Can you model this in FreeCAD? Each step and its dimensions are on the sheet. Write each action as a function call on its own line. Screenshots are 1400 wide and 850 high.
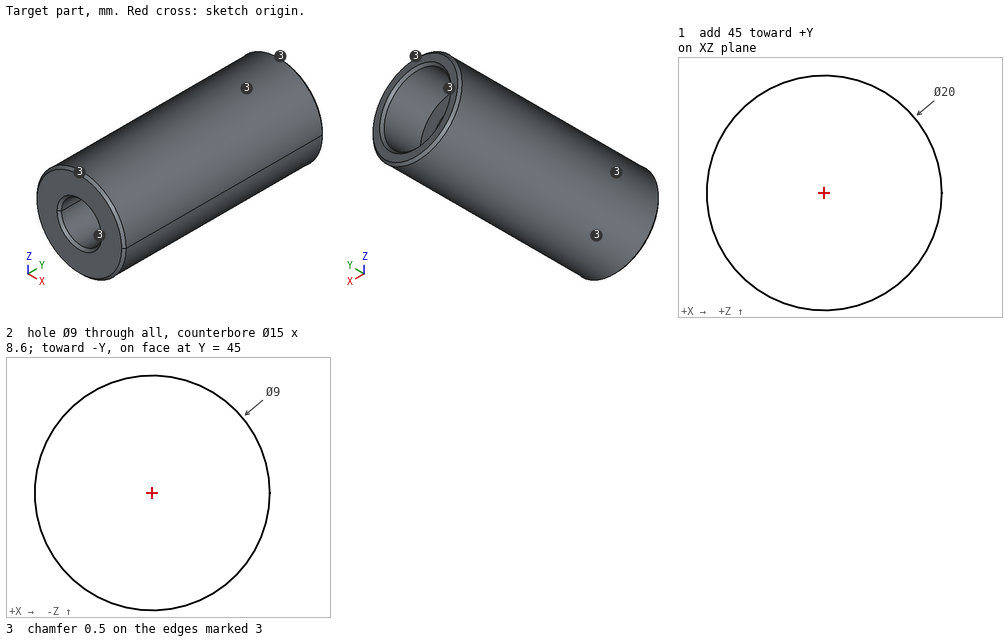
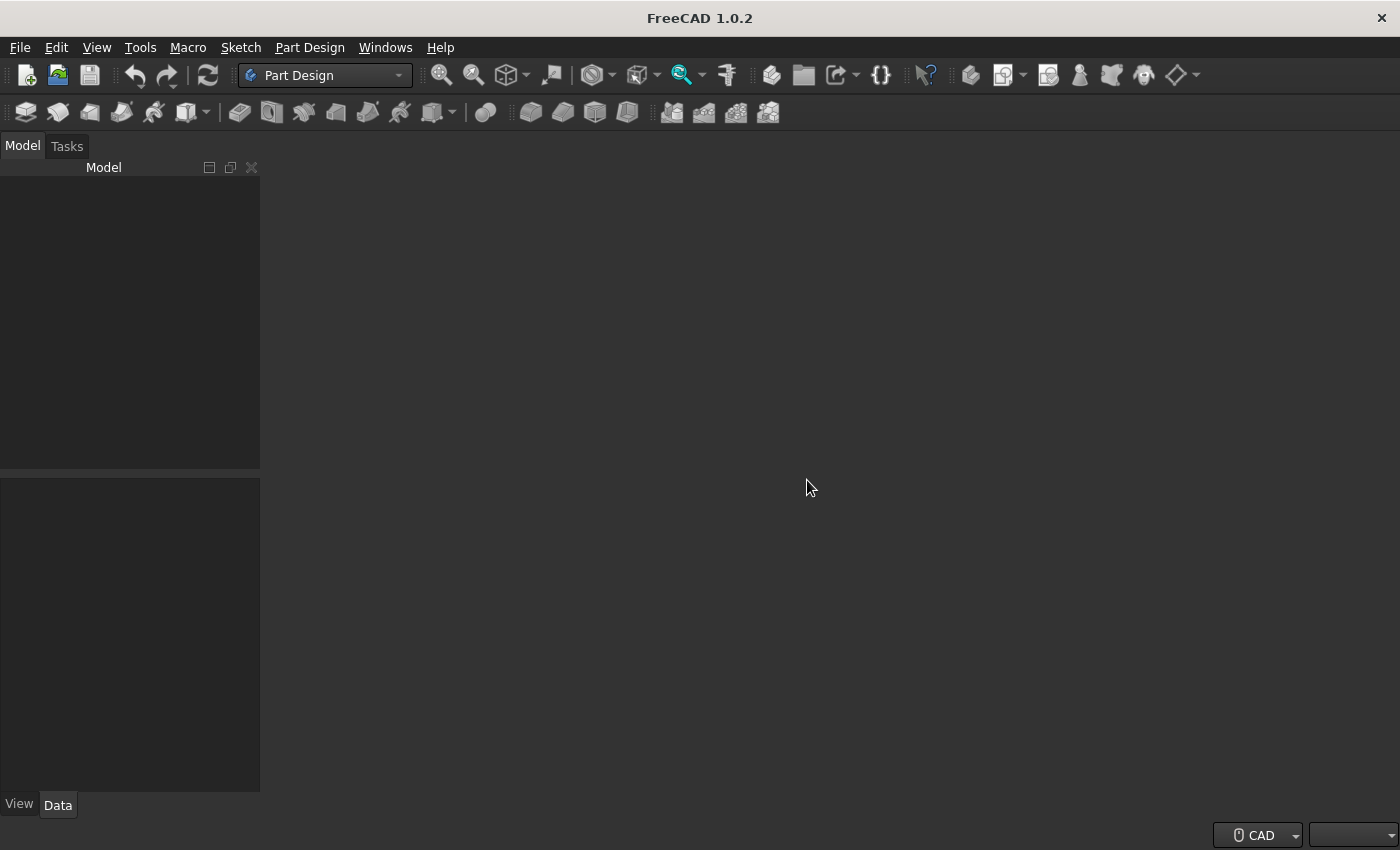
key(ctrl+n)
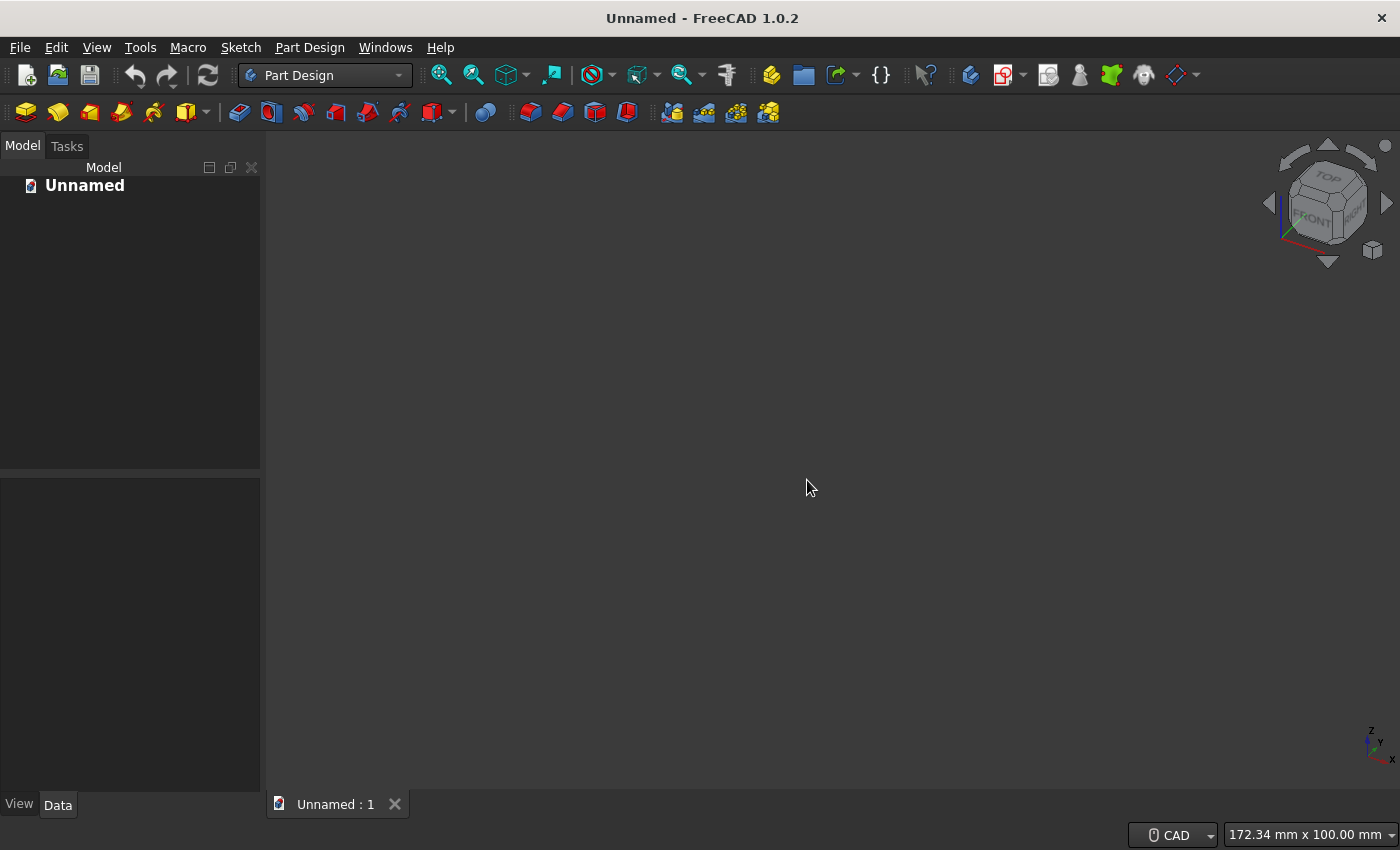
click(1004, 76)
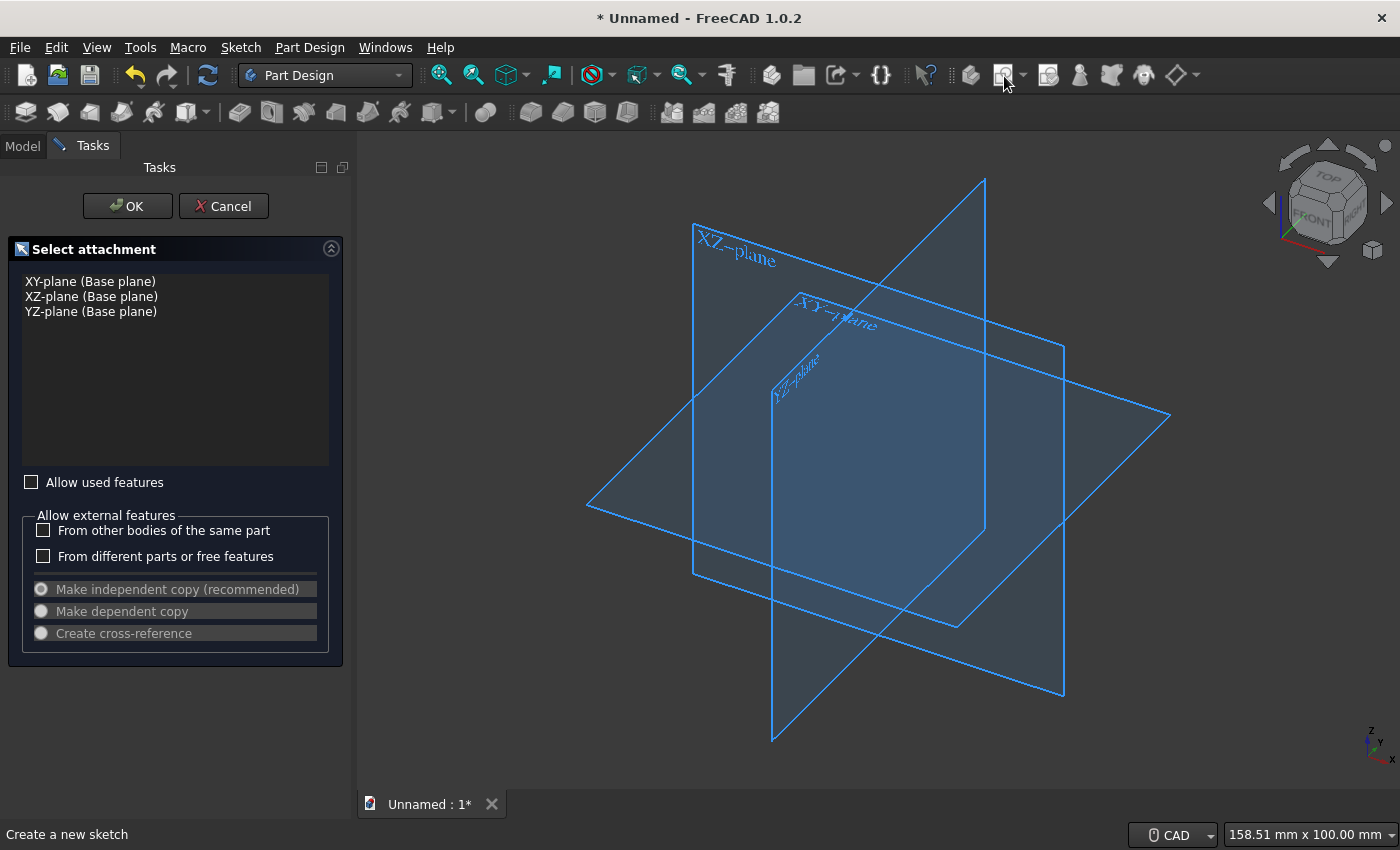
click(82, 296)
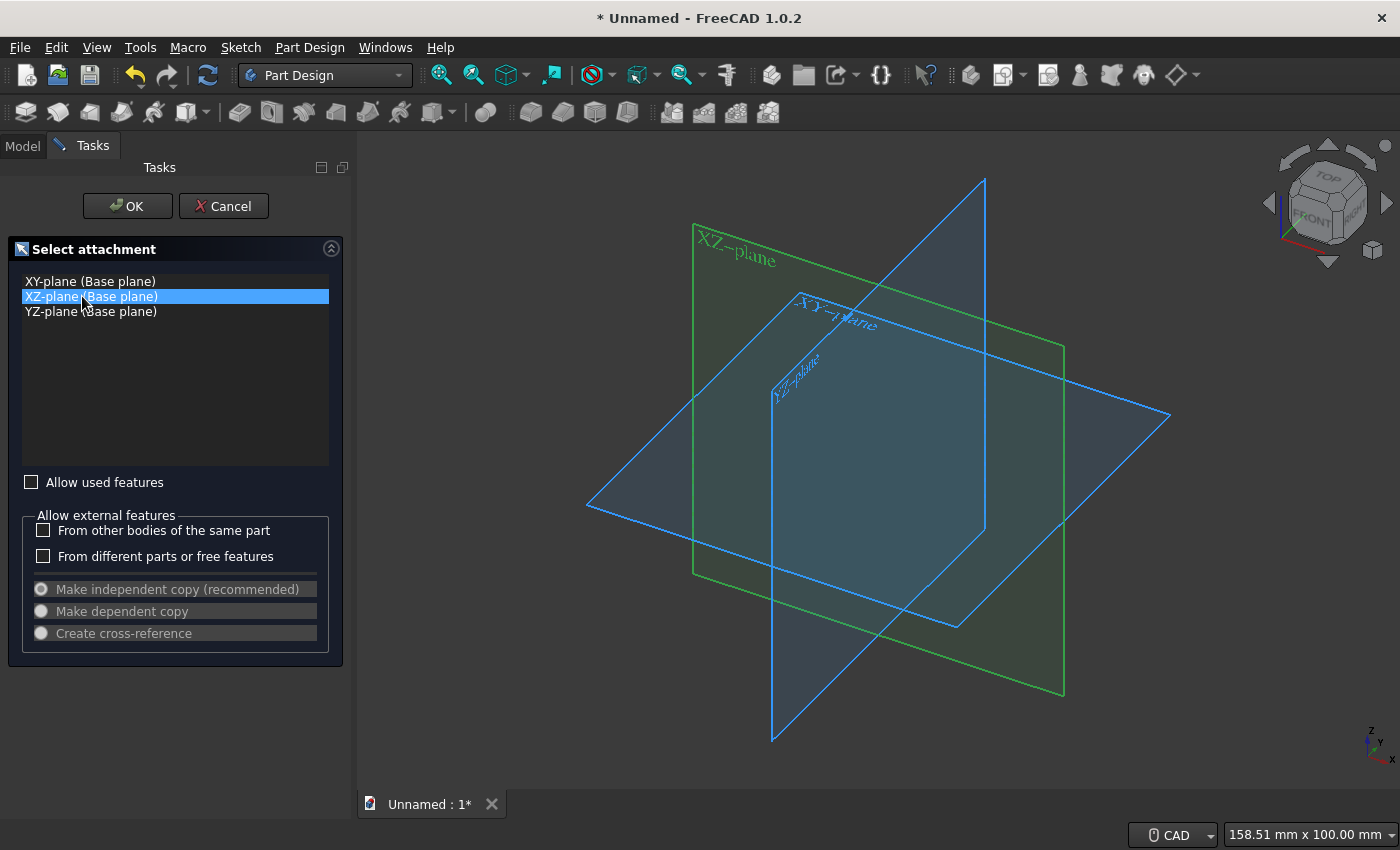
click(128, 206)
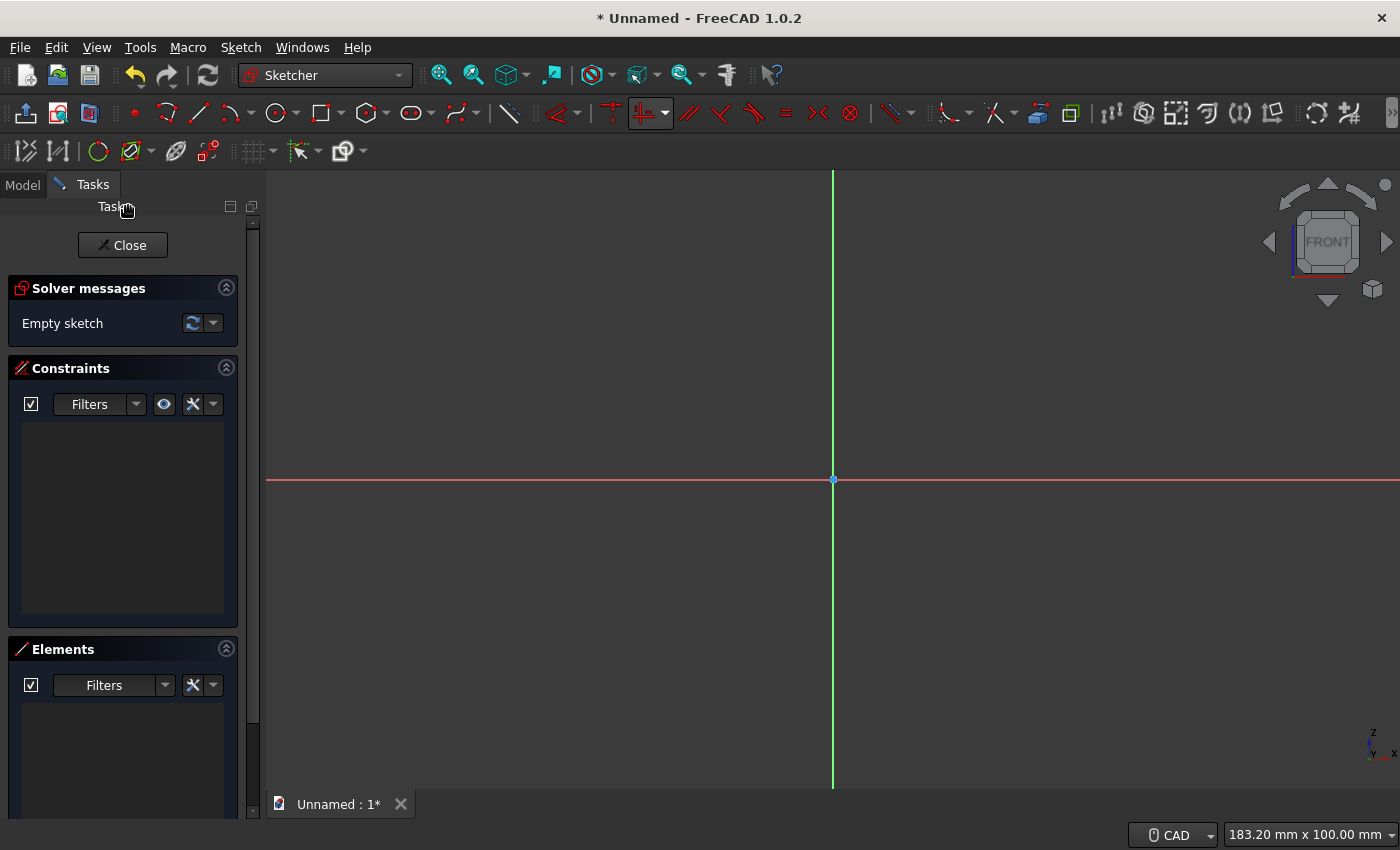
scroll(863, 480, up, 6)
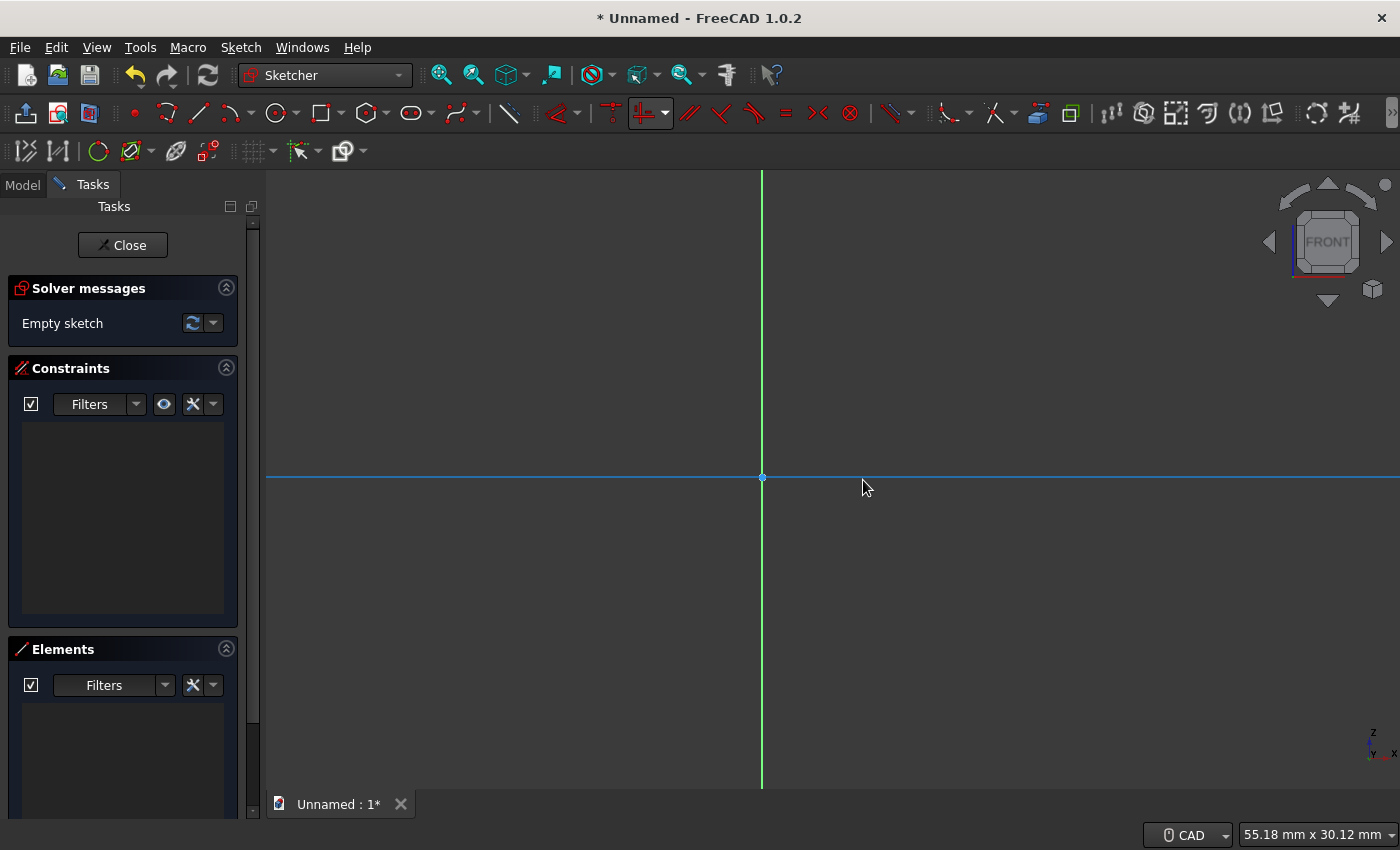
click(276, 114)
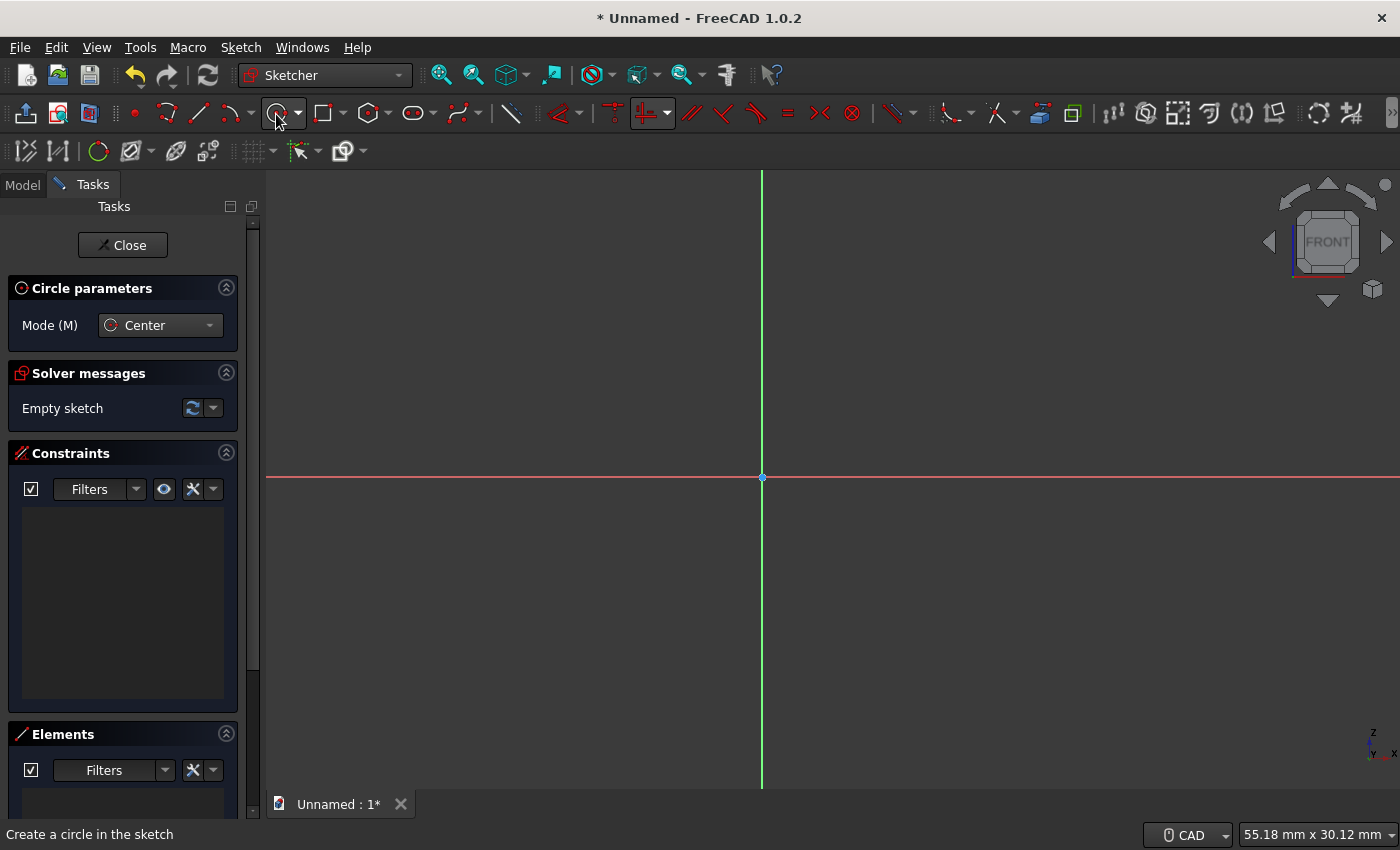
click(762, 477)
move(907, 332)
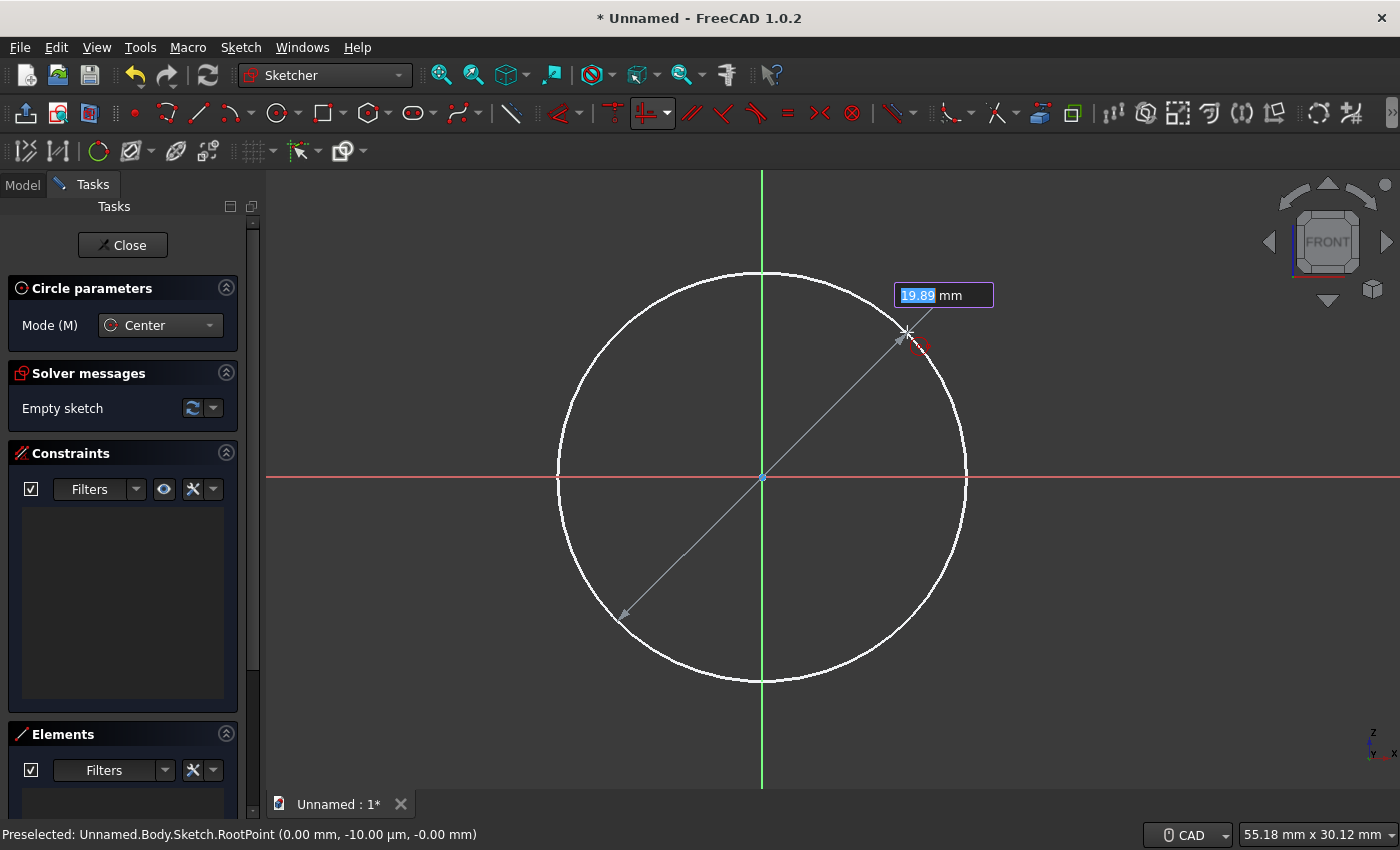
text(20)
key(Return)
key(Escape)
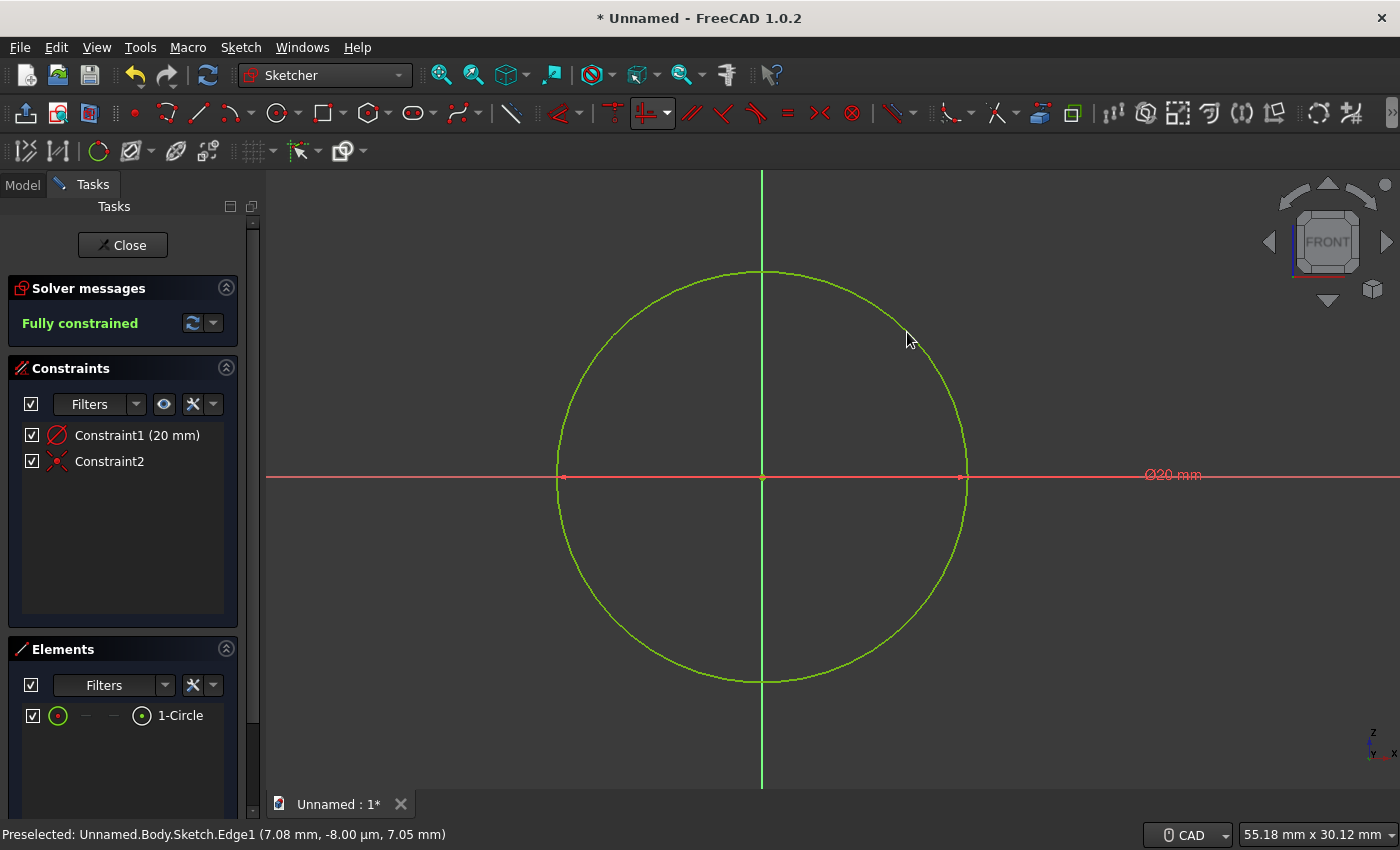
click(123, 245)